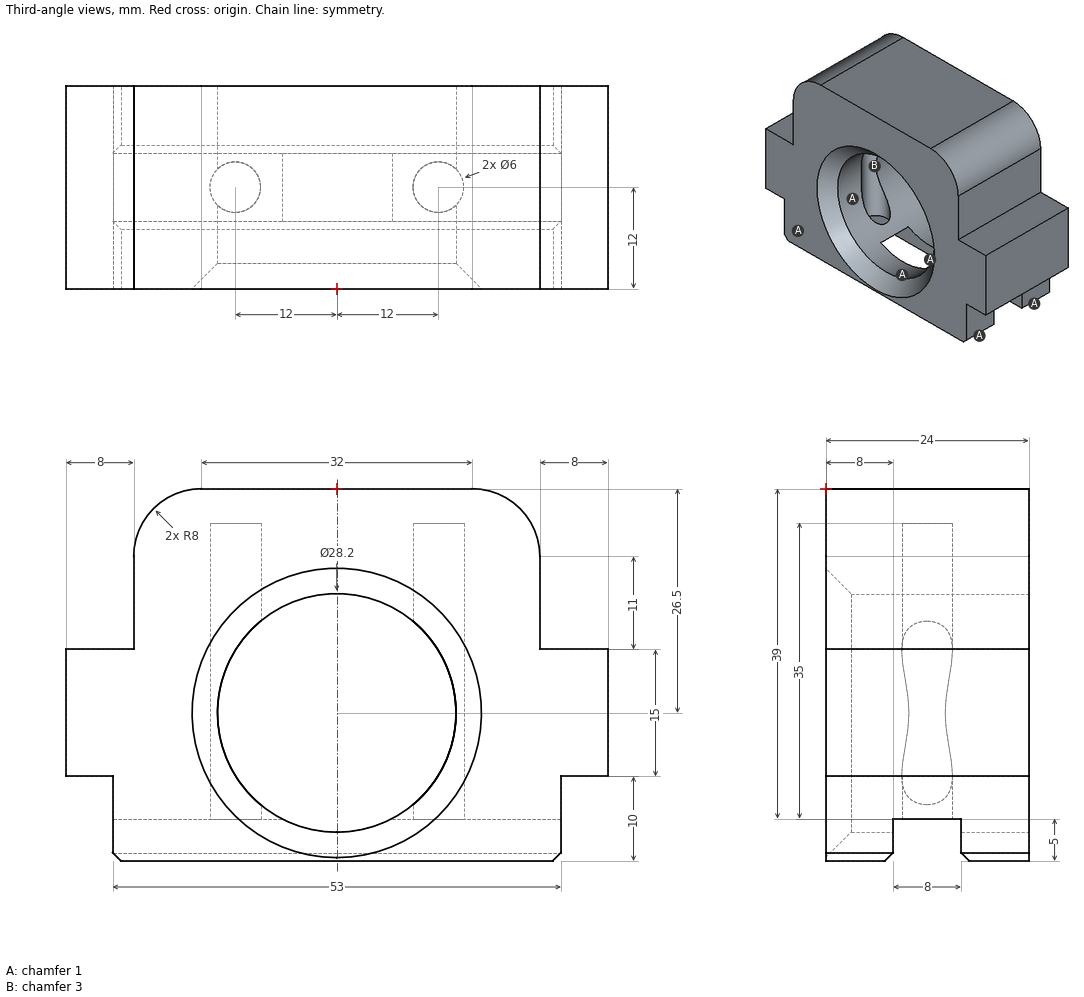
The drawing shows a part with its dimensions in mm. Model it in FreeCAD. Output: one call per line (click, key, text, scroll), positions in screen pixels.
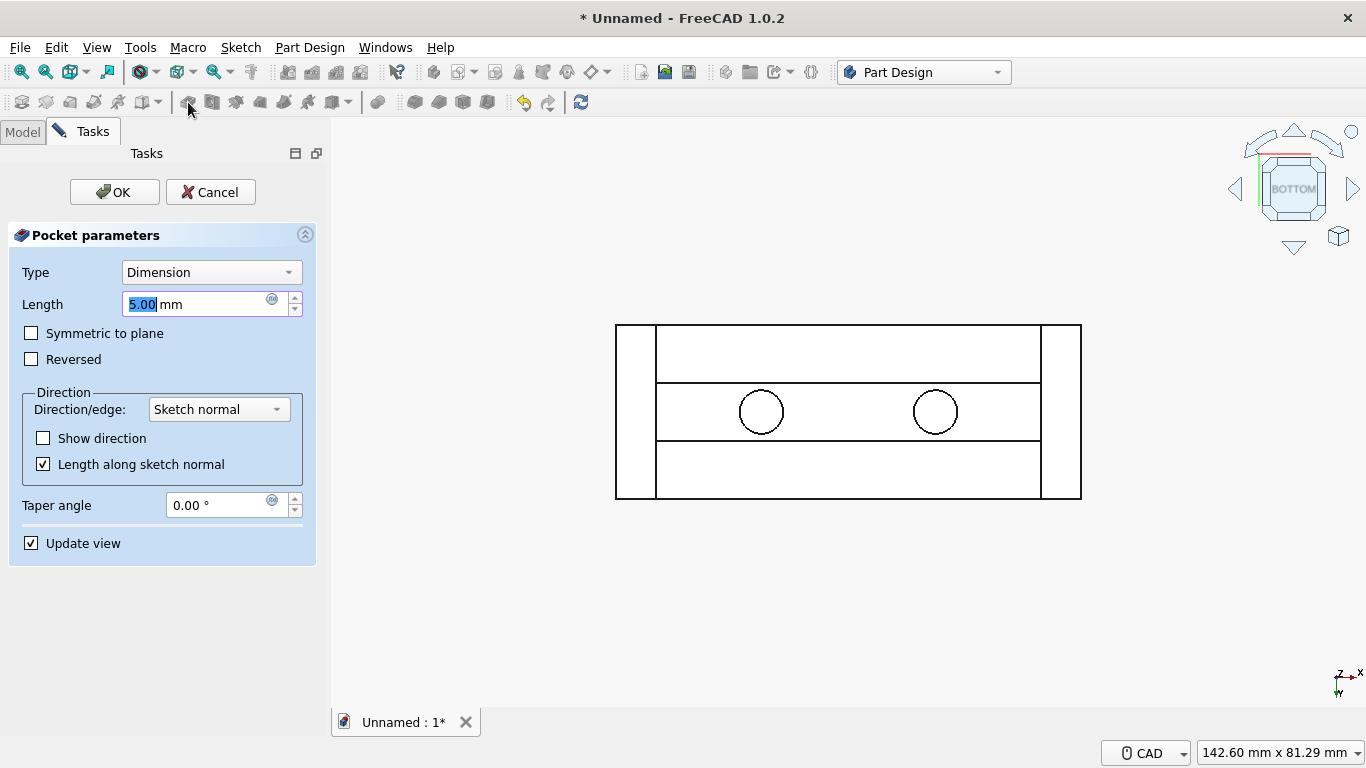
text(35)
key(Tab)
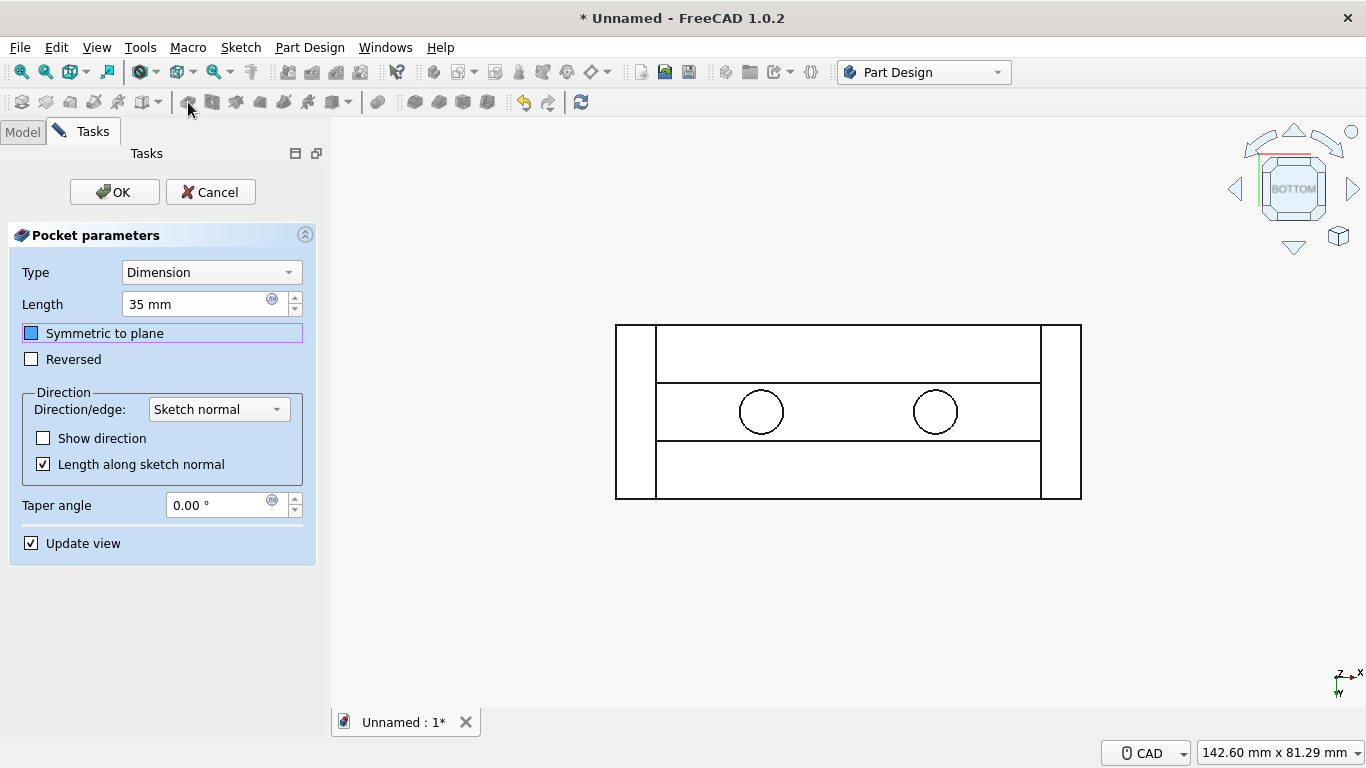
click(115, 192)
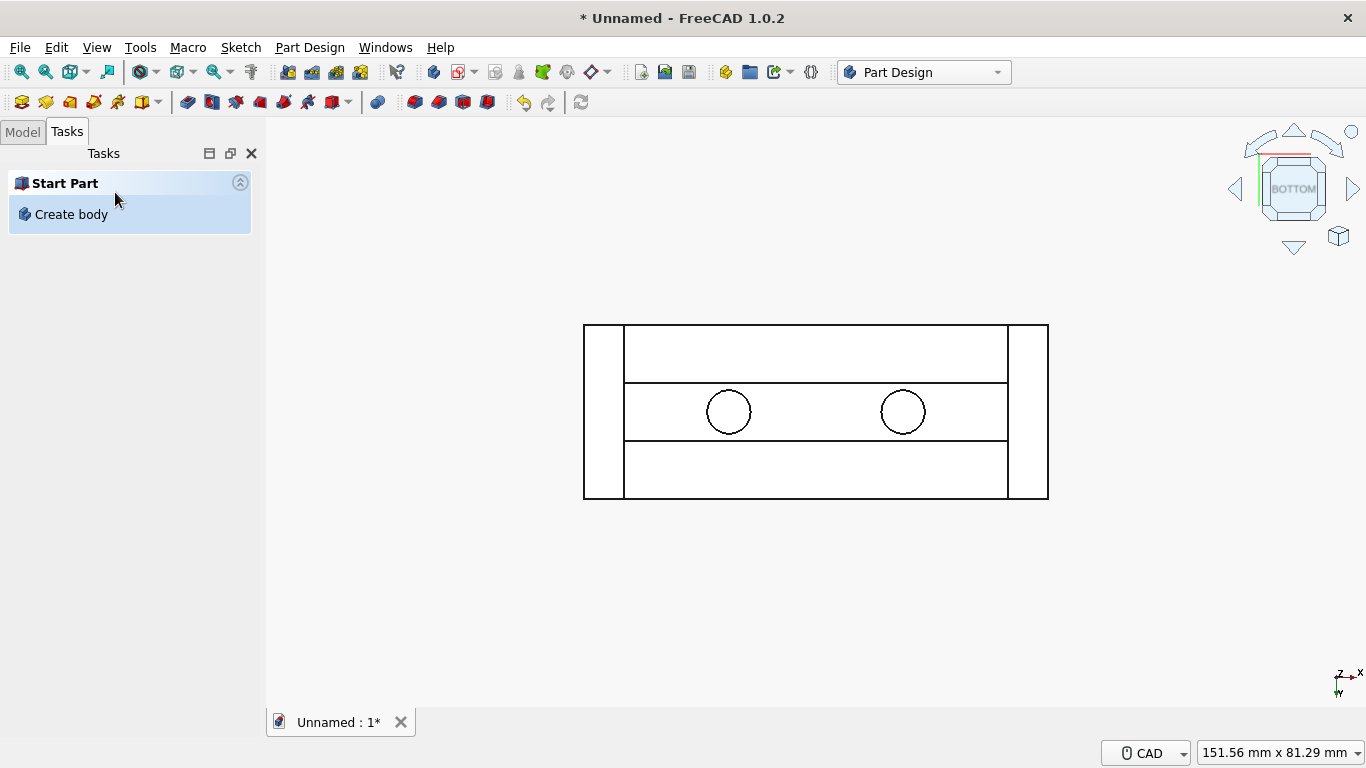
click(22, 72)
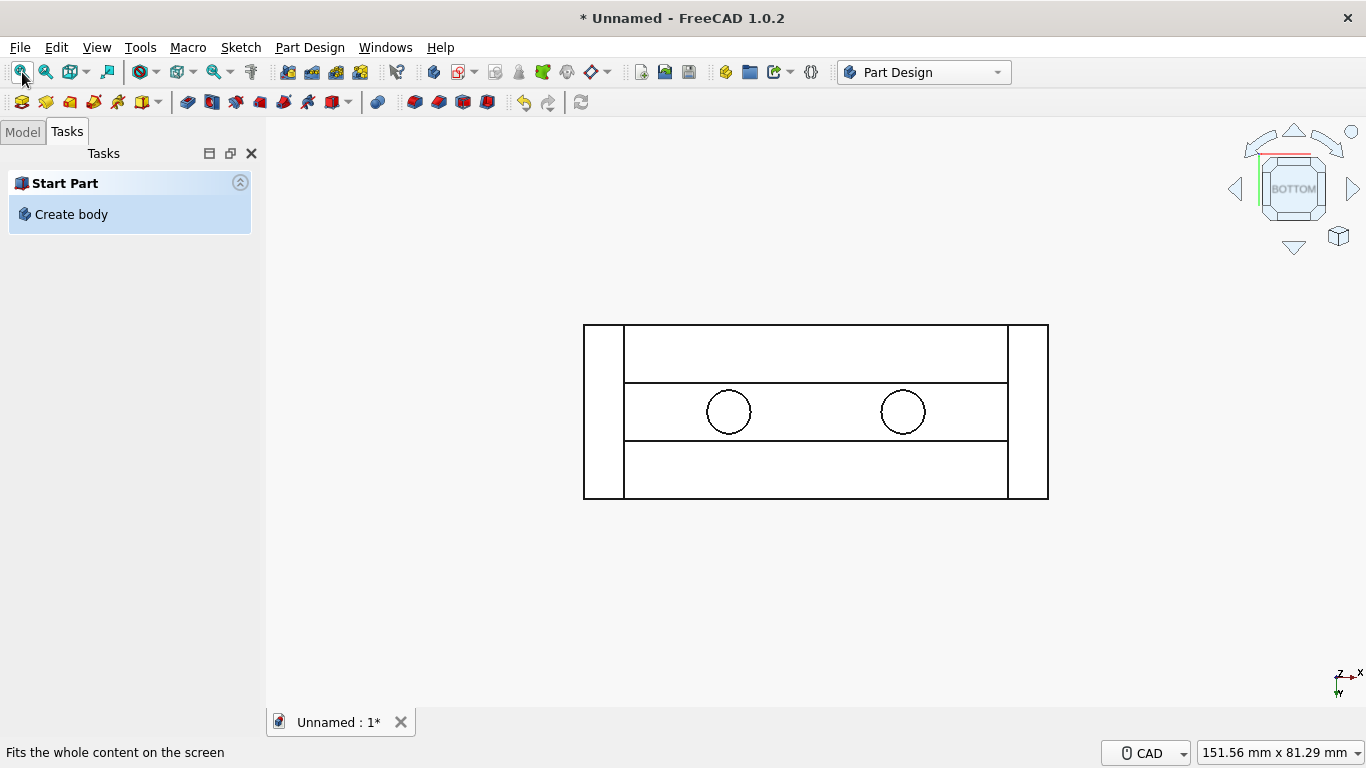
click(458, 72)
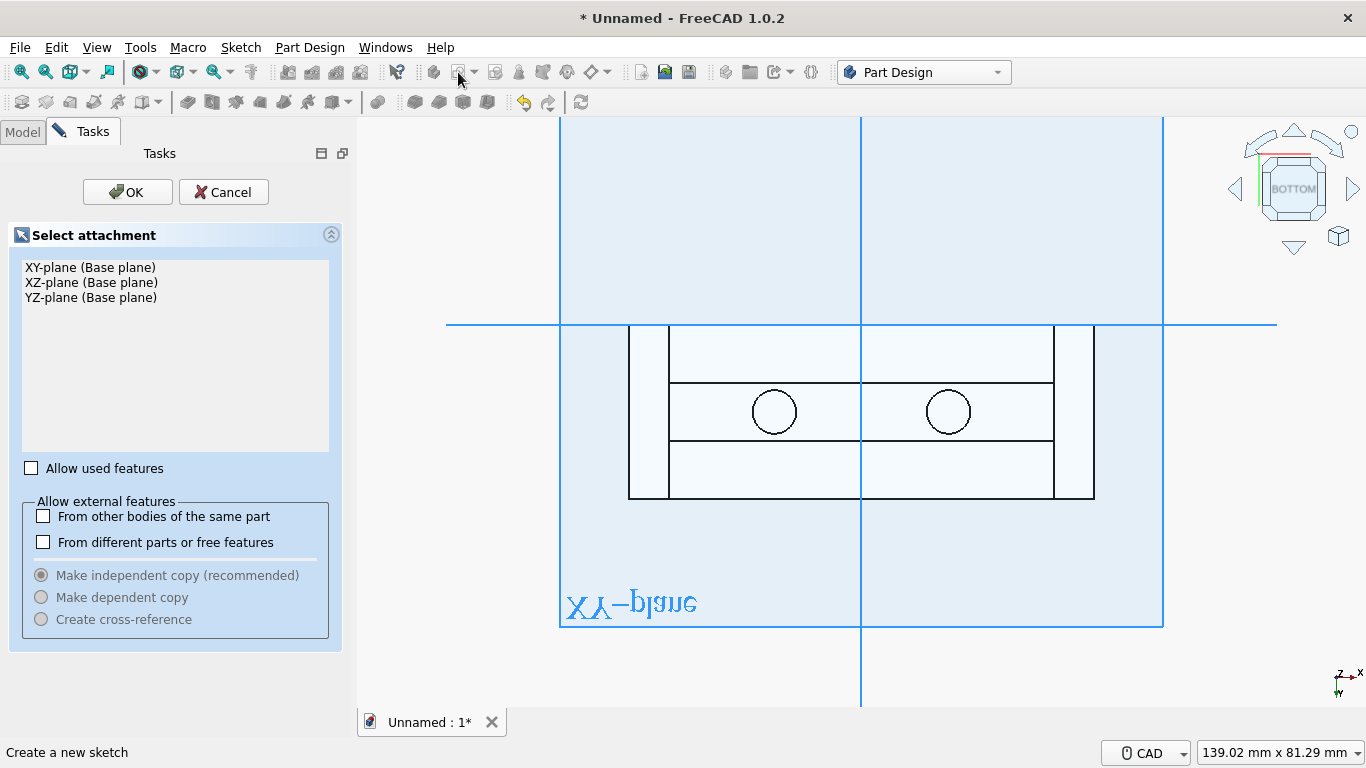
click(82, 282)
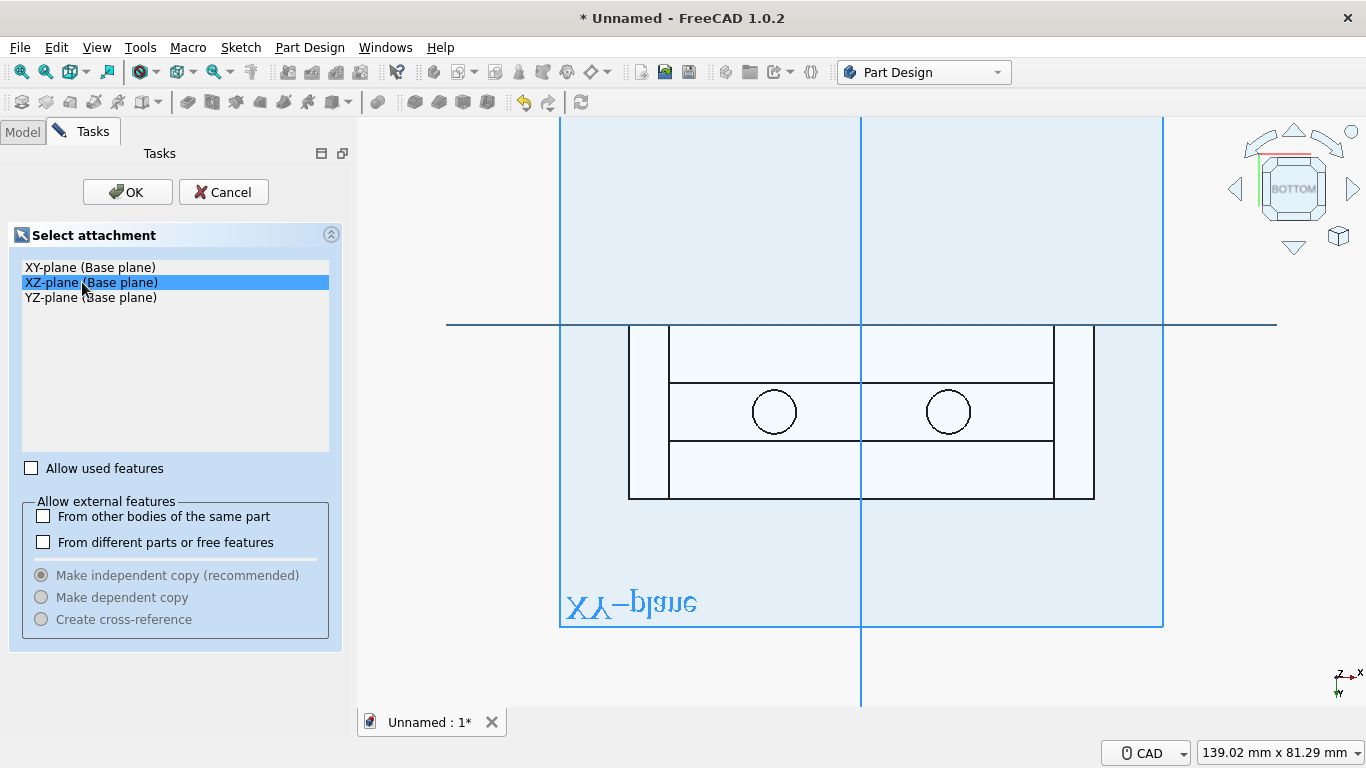
click(128, 192)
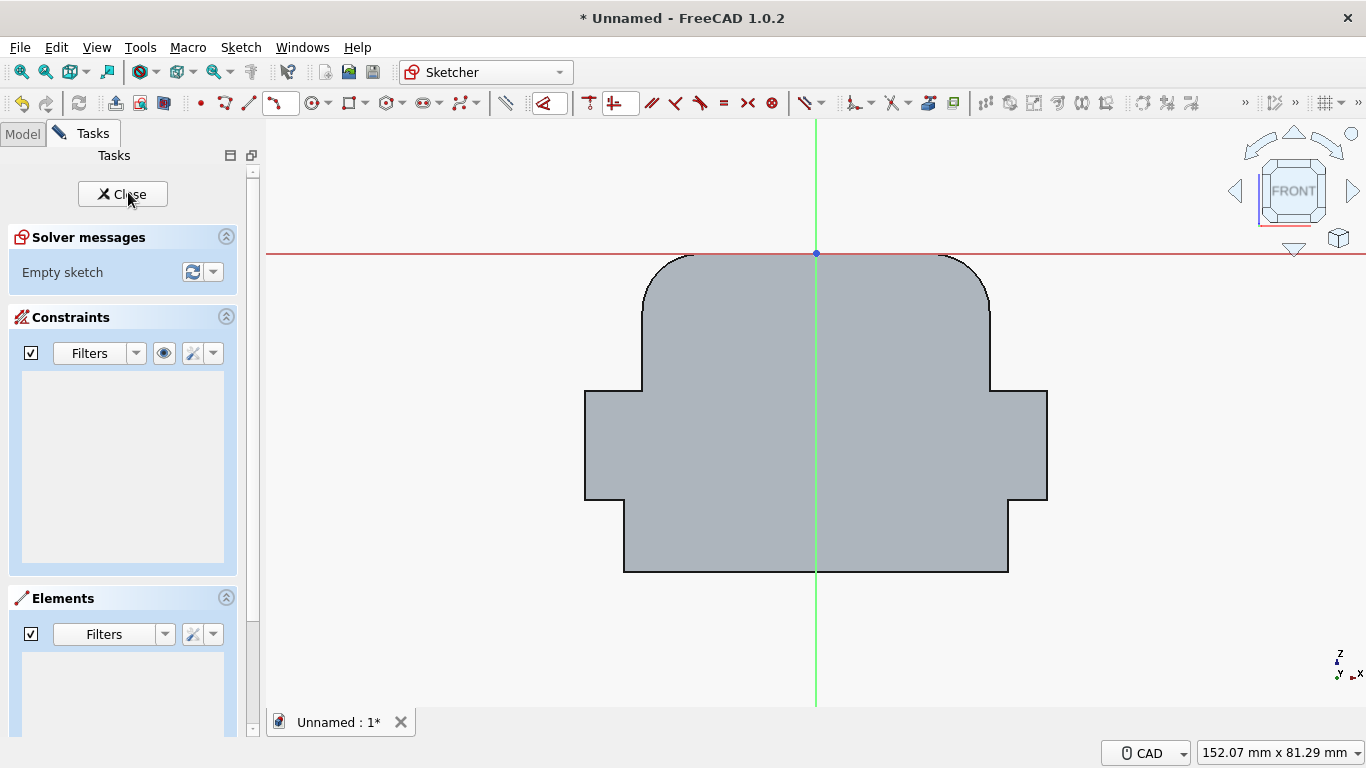
click(312, 104)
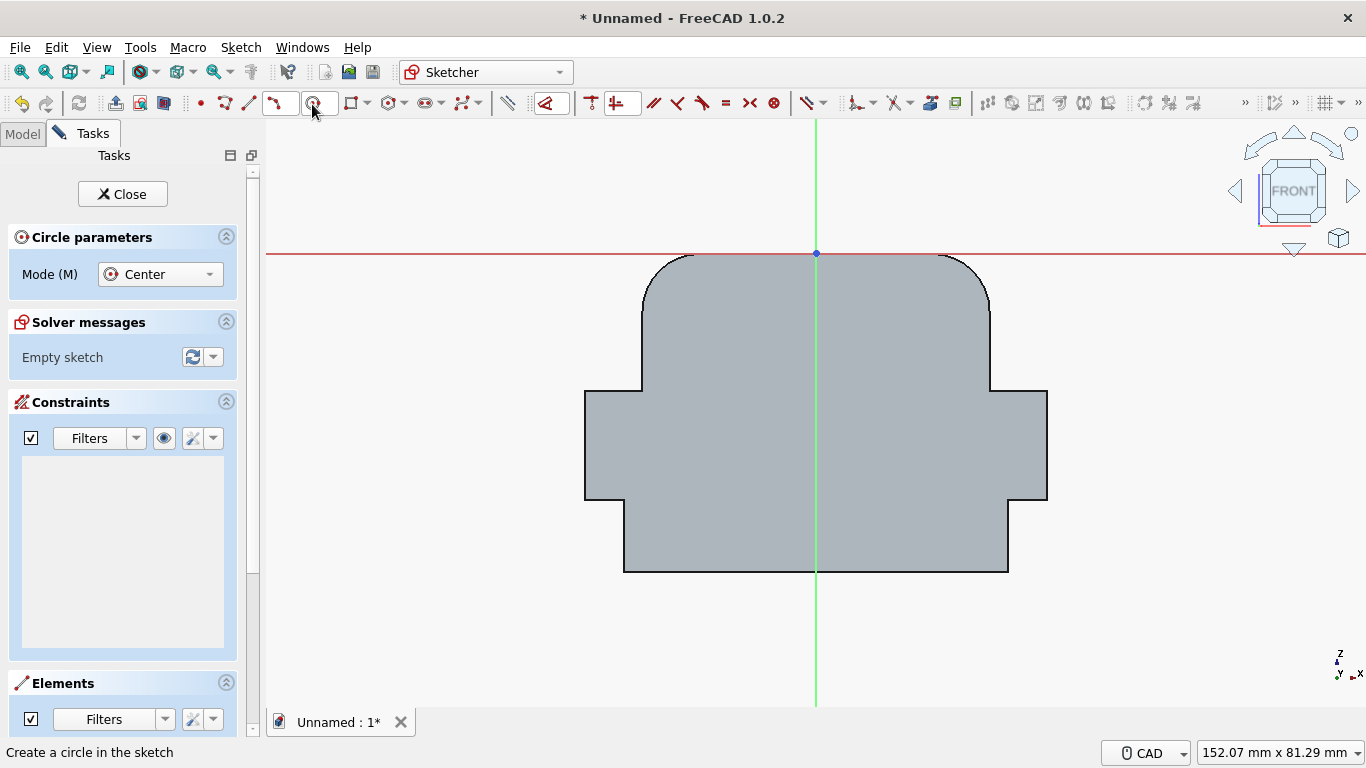
click(816, 446)
move(888, 373)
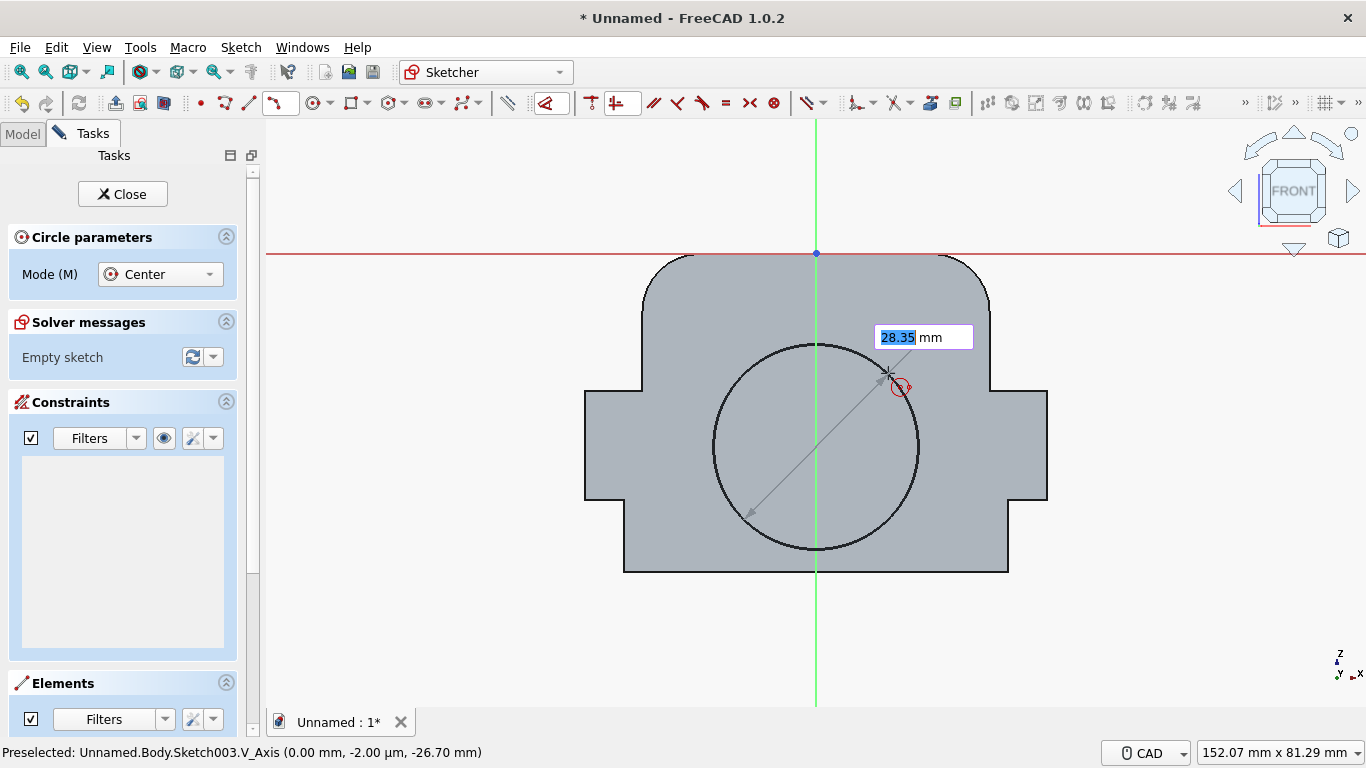
text(28.2)
key(Return)
key(Escape)